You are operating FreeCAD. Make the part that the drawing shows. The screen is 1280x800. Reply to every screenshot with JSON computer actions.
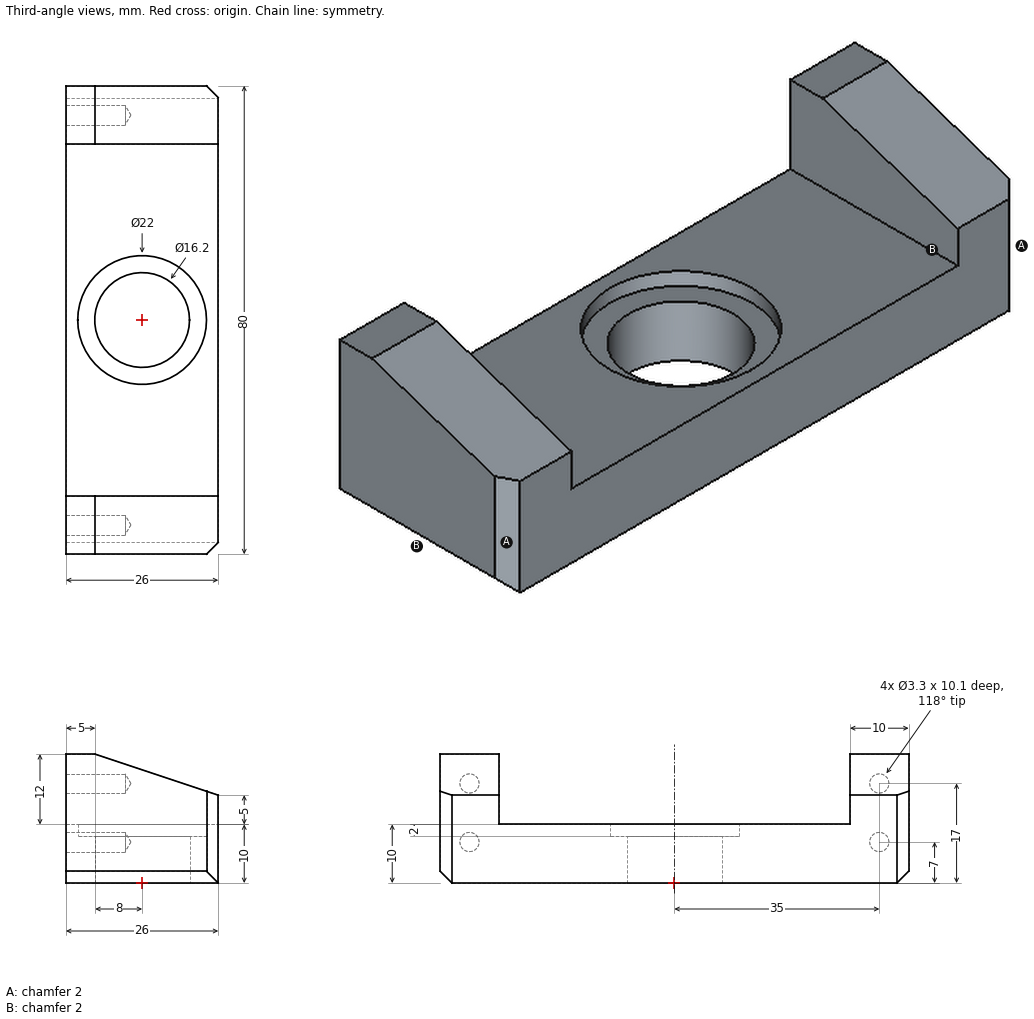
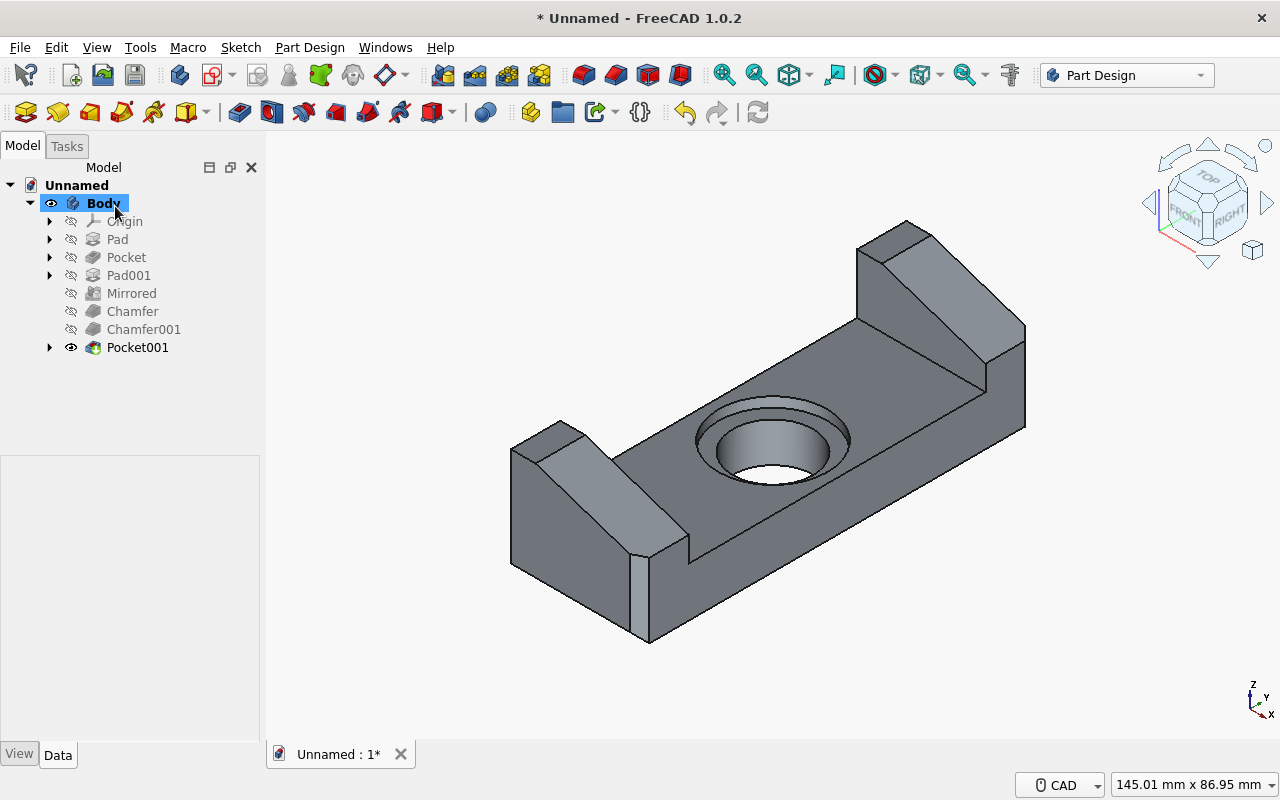
{"action": "key", "text": "6"}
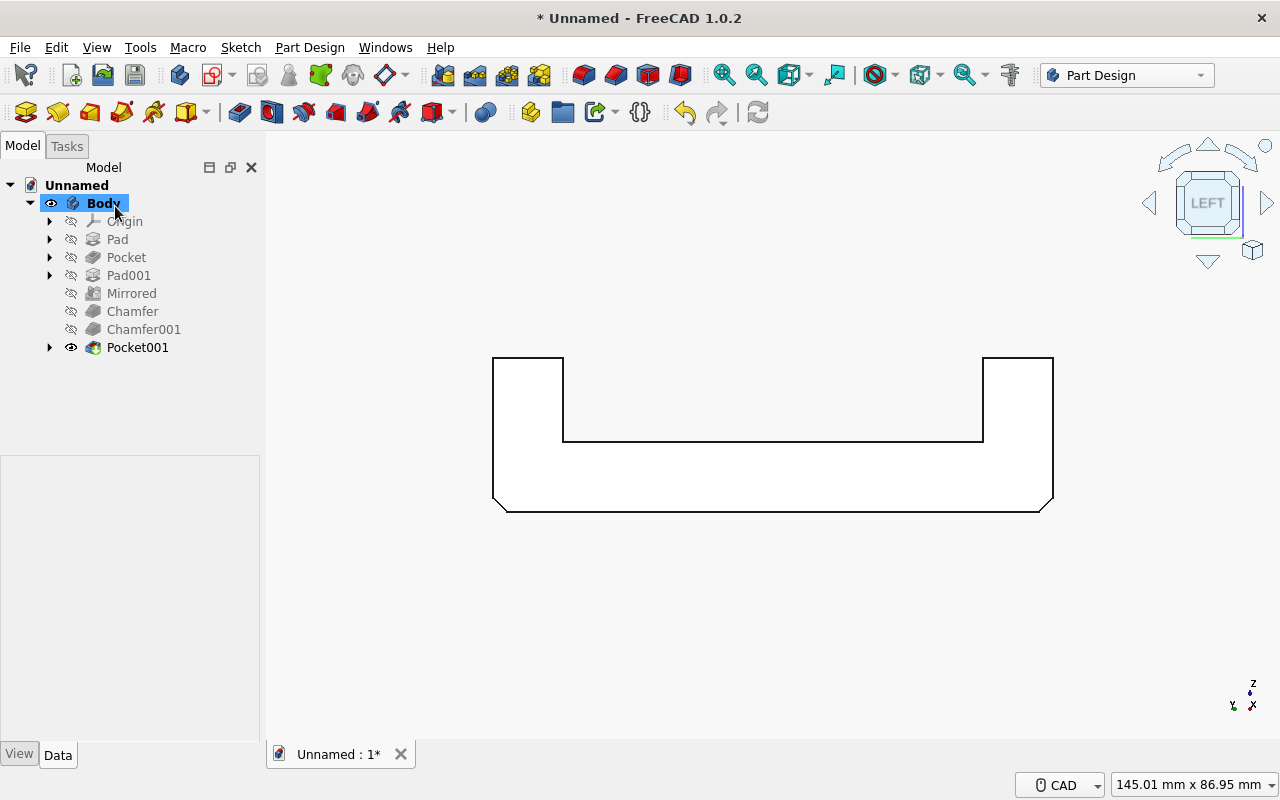
{"action": "left_click", "coordinate": [1013, 456]}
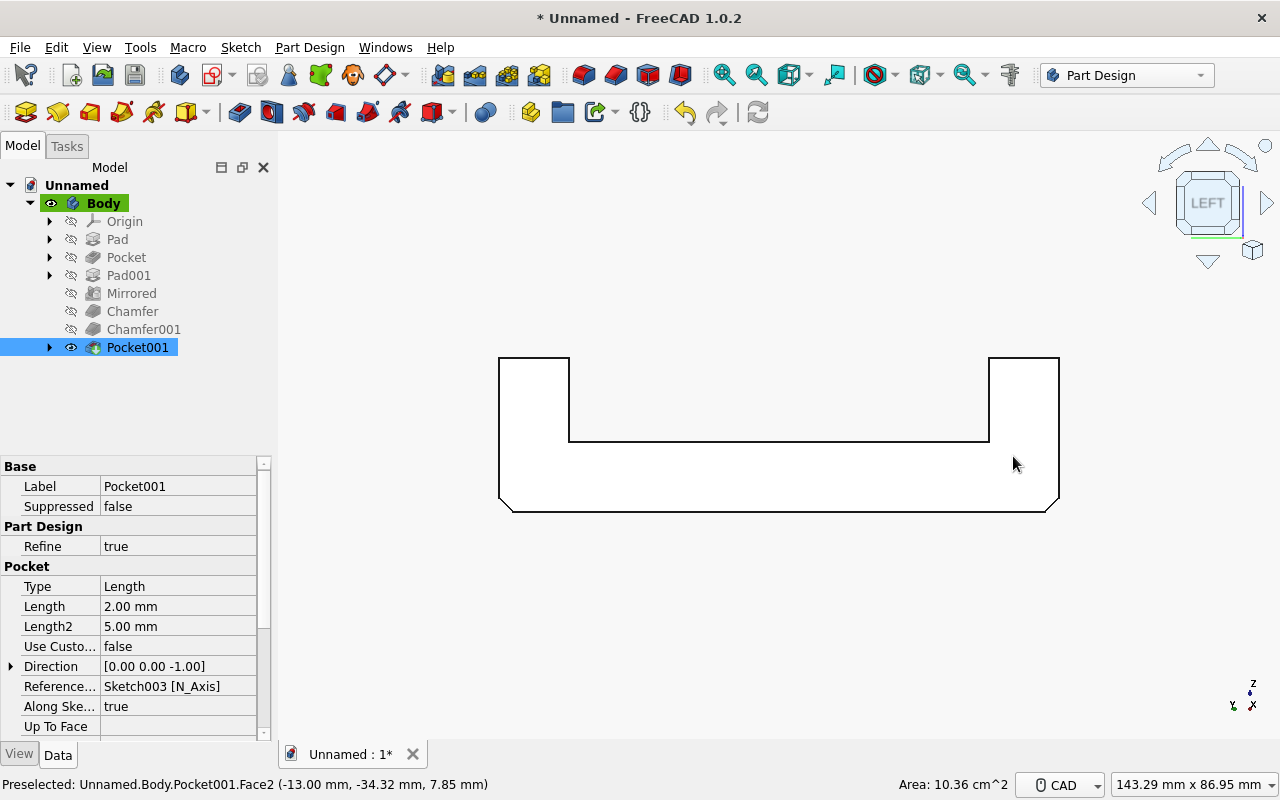
{"action": "left_click", "coordinate": [212, 76]}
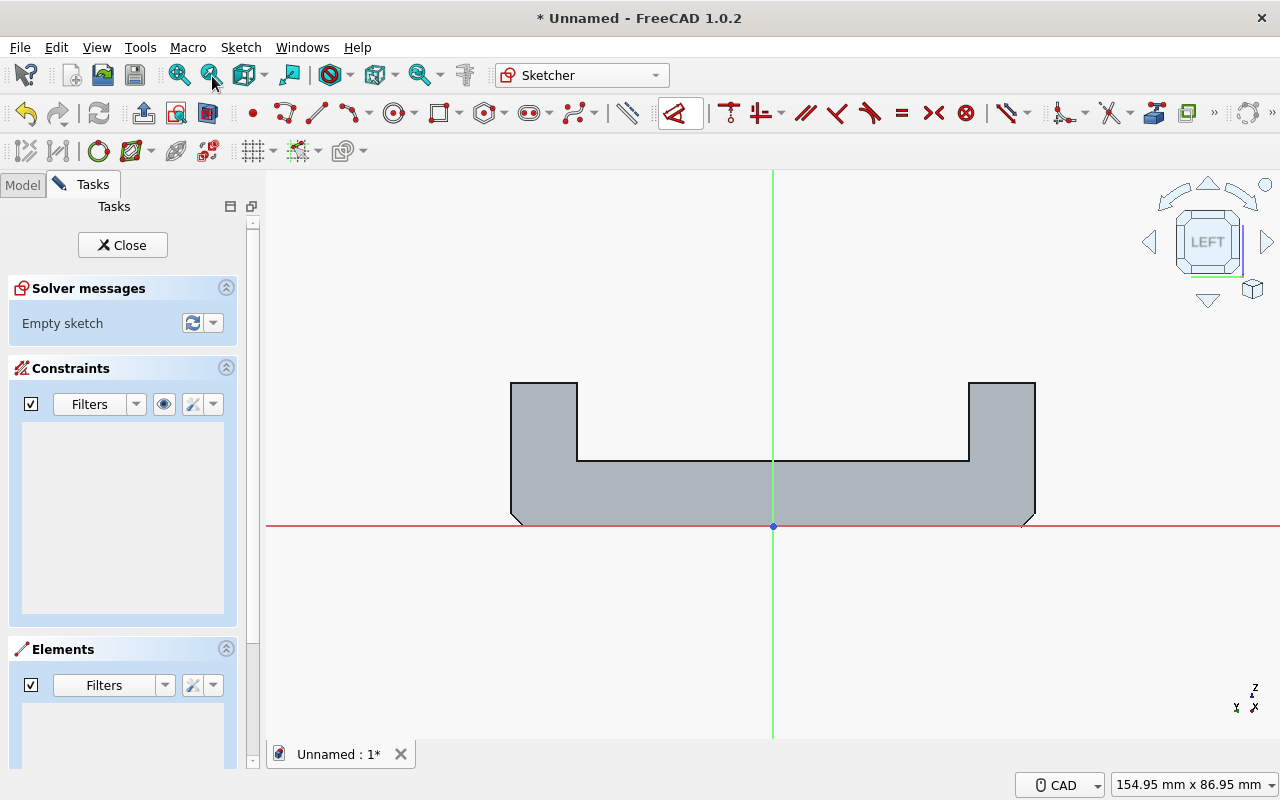
{"action": "left_click", "coordinate": [394, 114]}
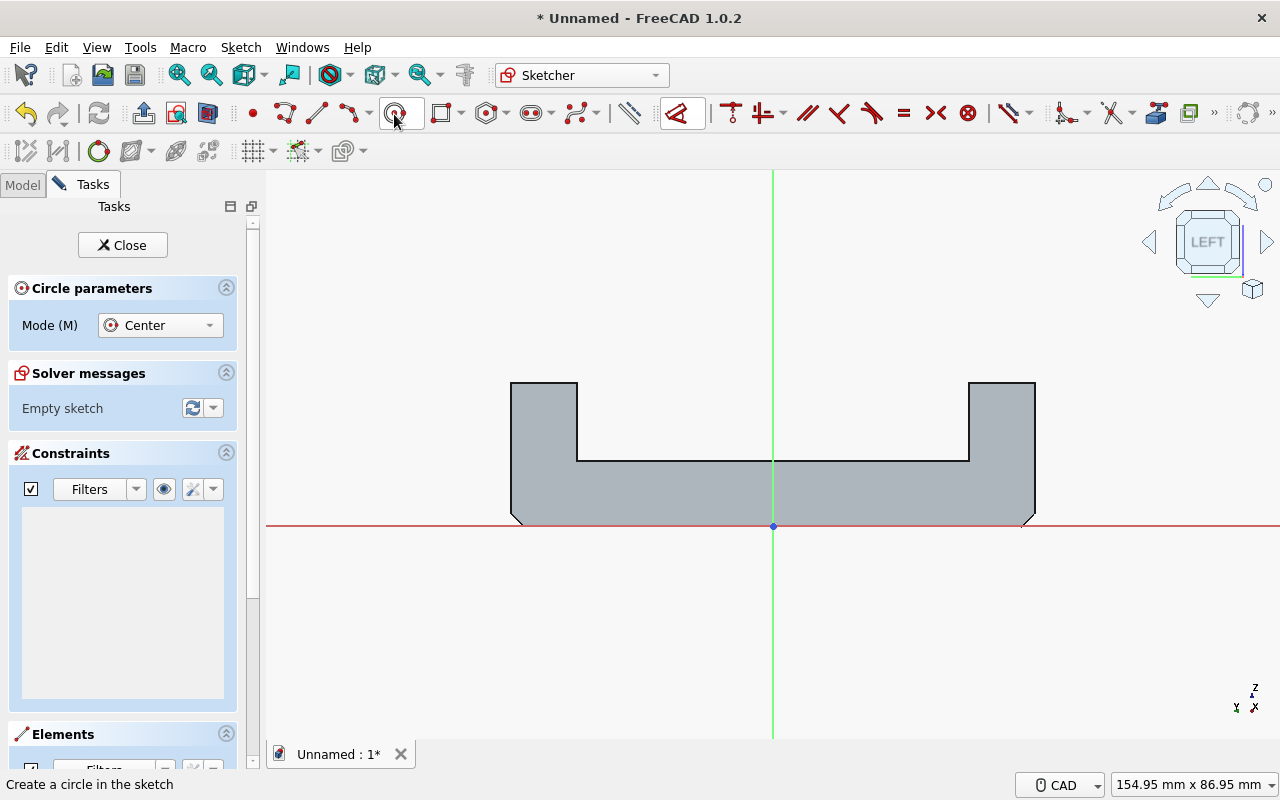
{"action": "scroll", "coordinate": [544, 415], "scroll_direction": "up", "scroll_amount": 4}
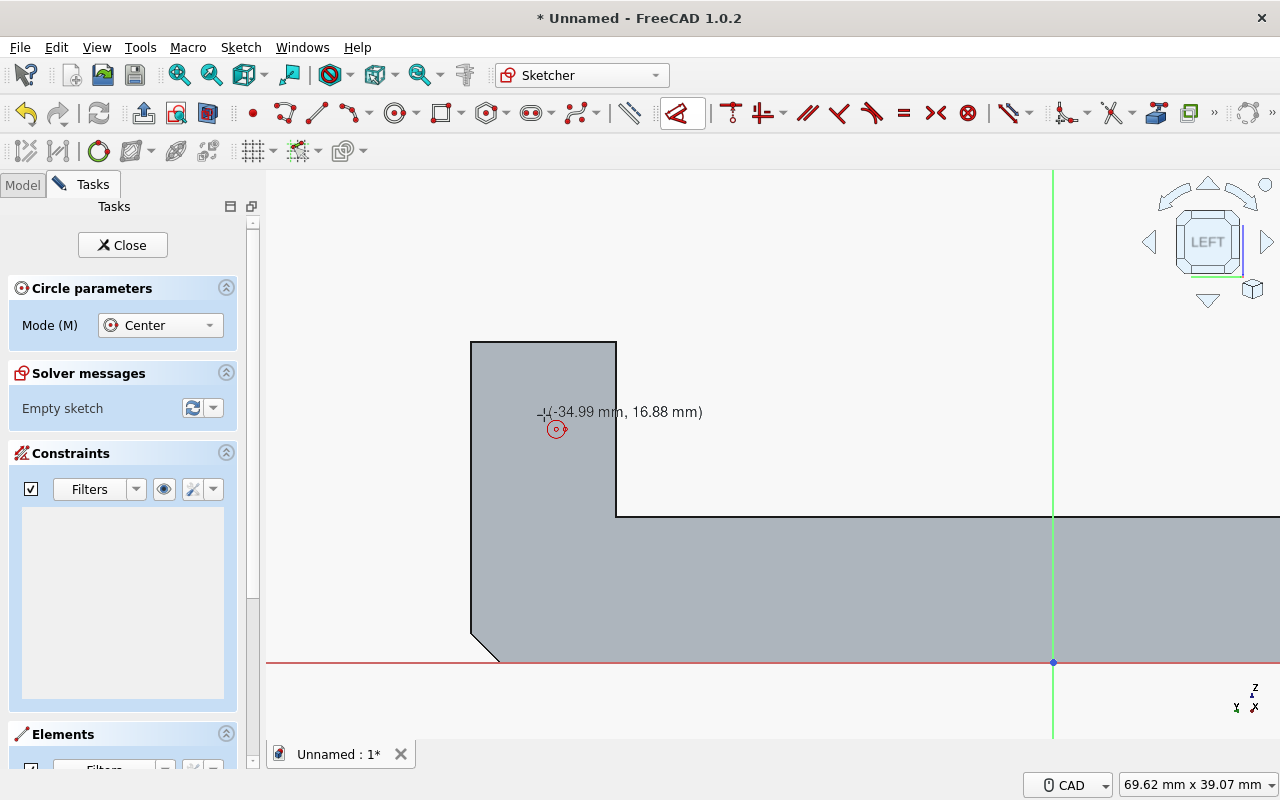
{"action": "left_click", "coordinate": [544, 415]}
{"action": "left_click", "coordinate": [561, 398]}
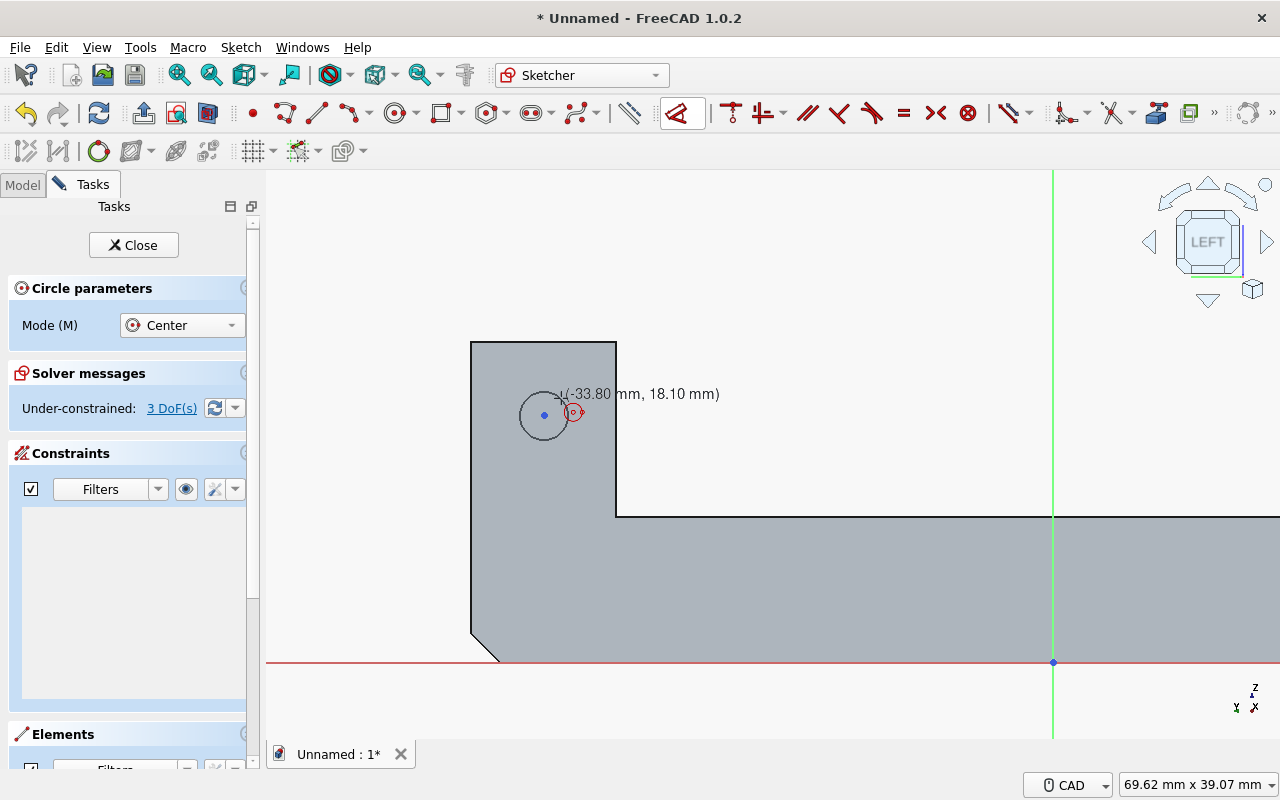
{"action": "left_click", "coordinate": [544, 561]}
{"action": "left_click", "coordinate": [561, 544]}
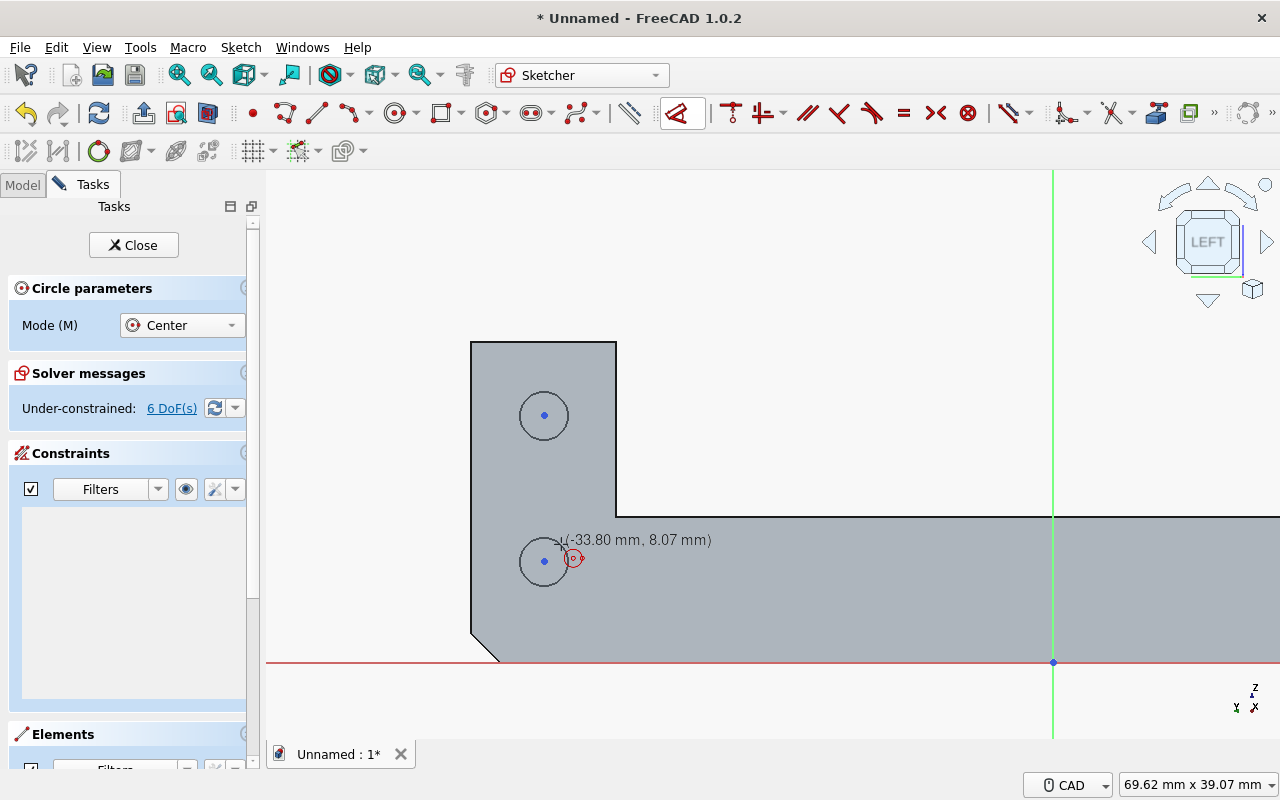
{"action": "scroll", "coordinate": [294, 367], "scroll_direction": "down", "scroll_amount": 3}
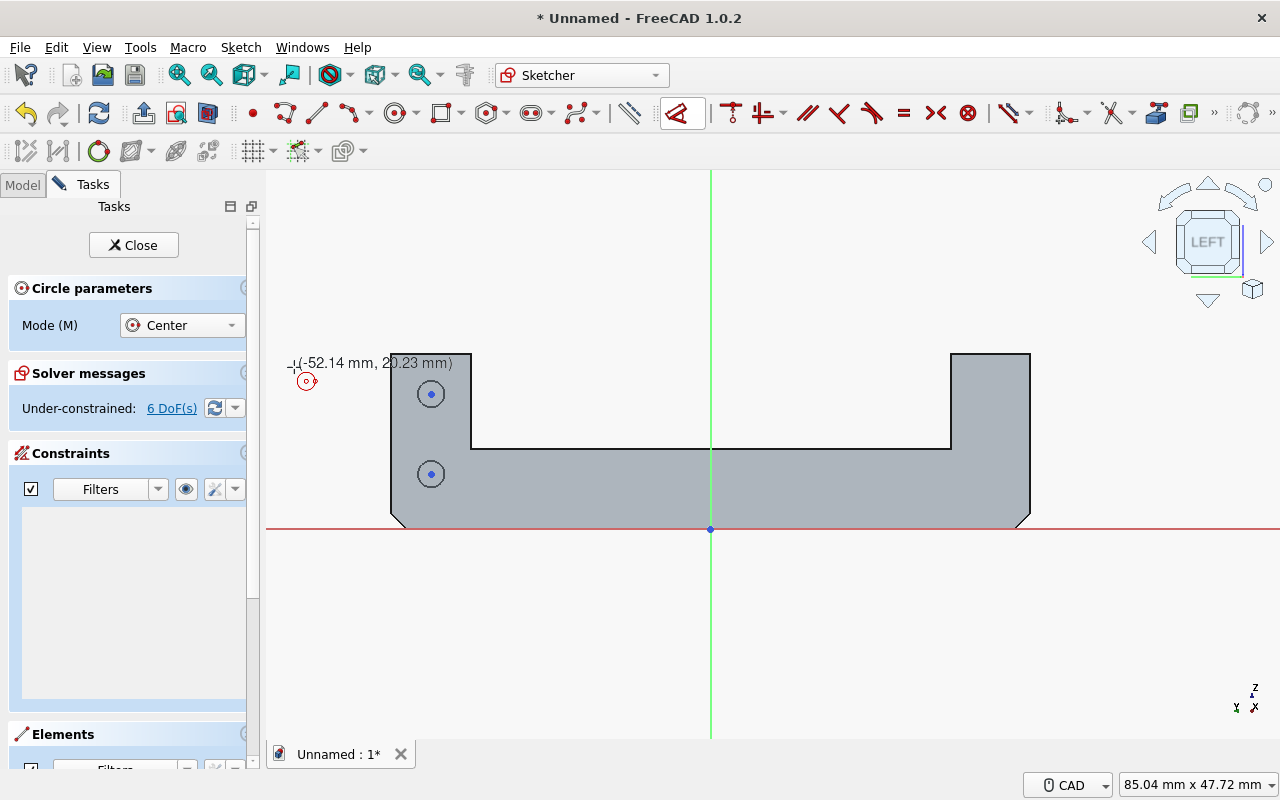
{"action": "scroll", "coordinate": [990, 473], "scroll_direction": "up", "scroll_amount": 3}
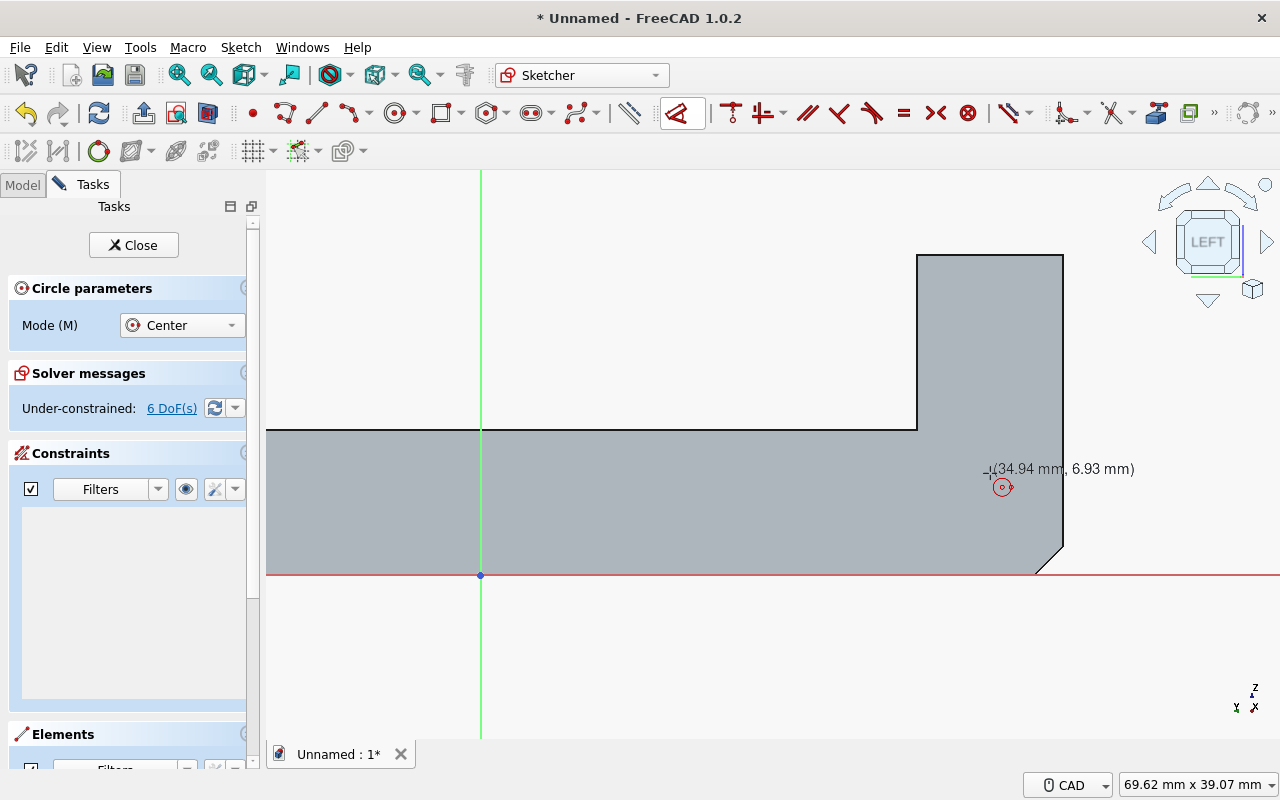
{"action": "left_click", "coordinate": [990, 473]}
{"action": "left_click", "coordinate": [1007, 456]}